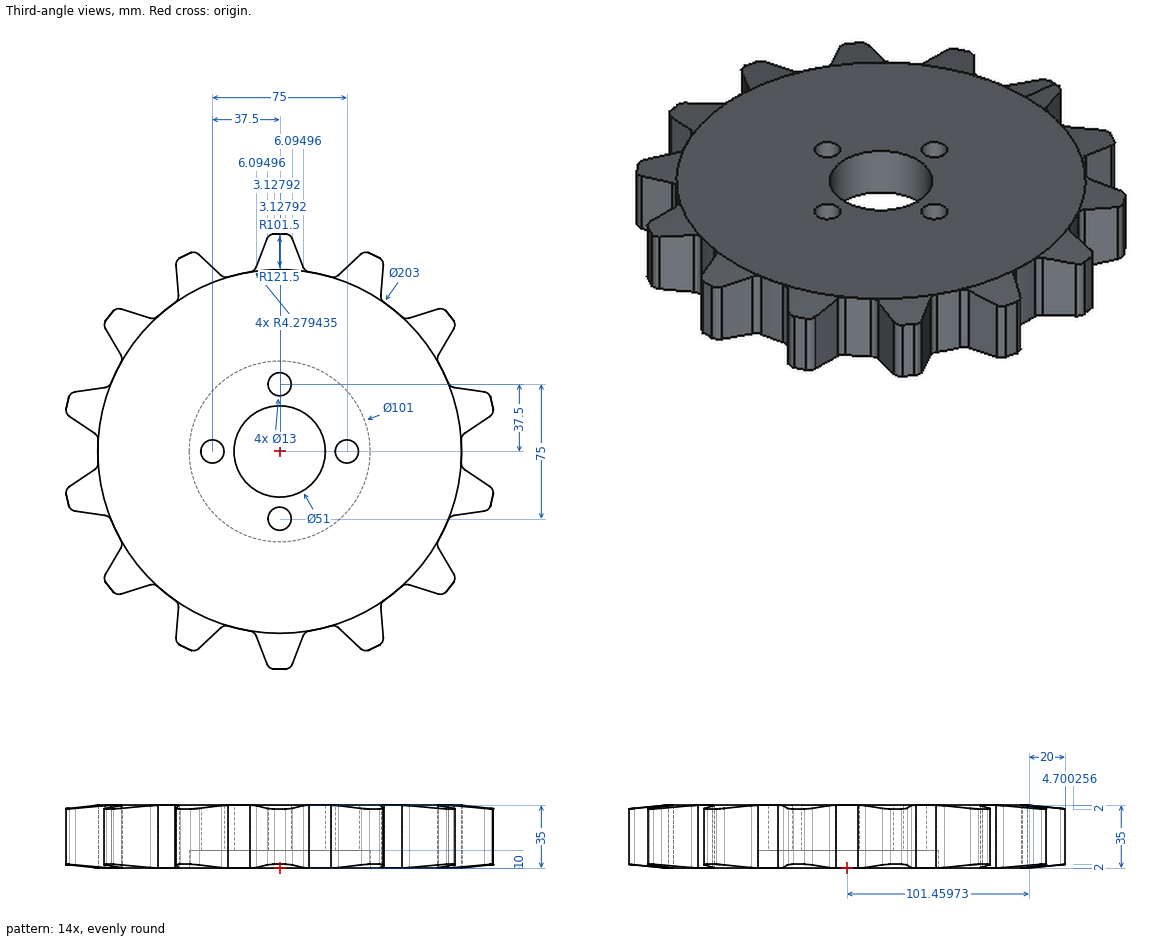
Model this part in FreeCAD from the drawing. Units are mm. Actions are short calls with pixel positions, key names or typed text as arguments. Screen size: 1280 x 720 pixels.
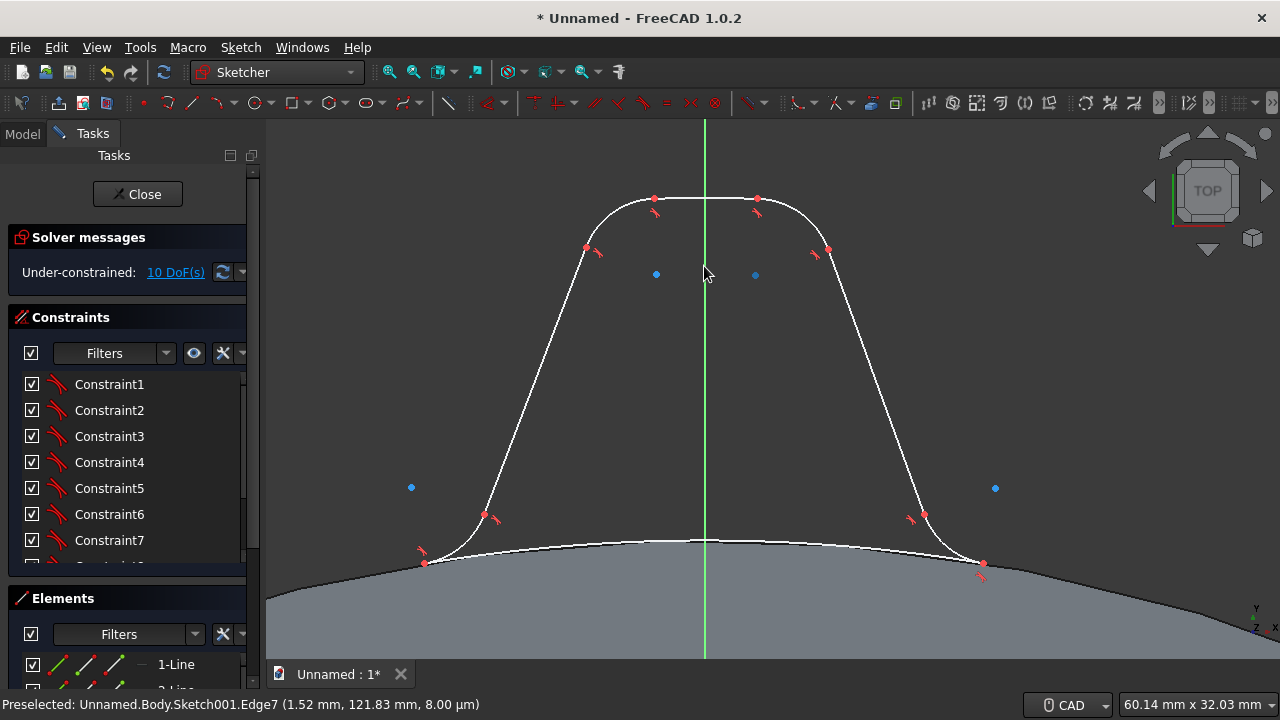
click(472, 536)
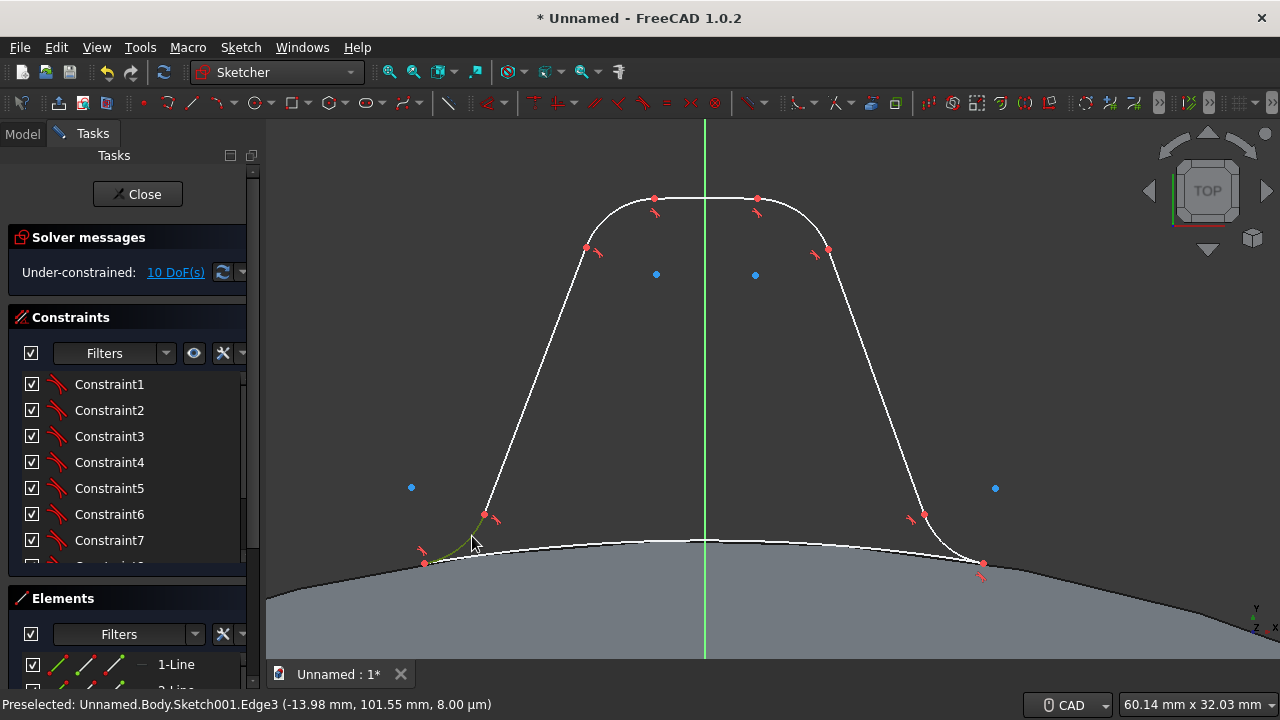
click(936, 535)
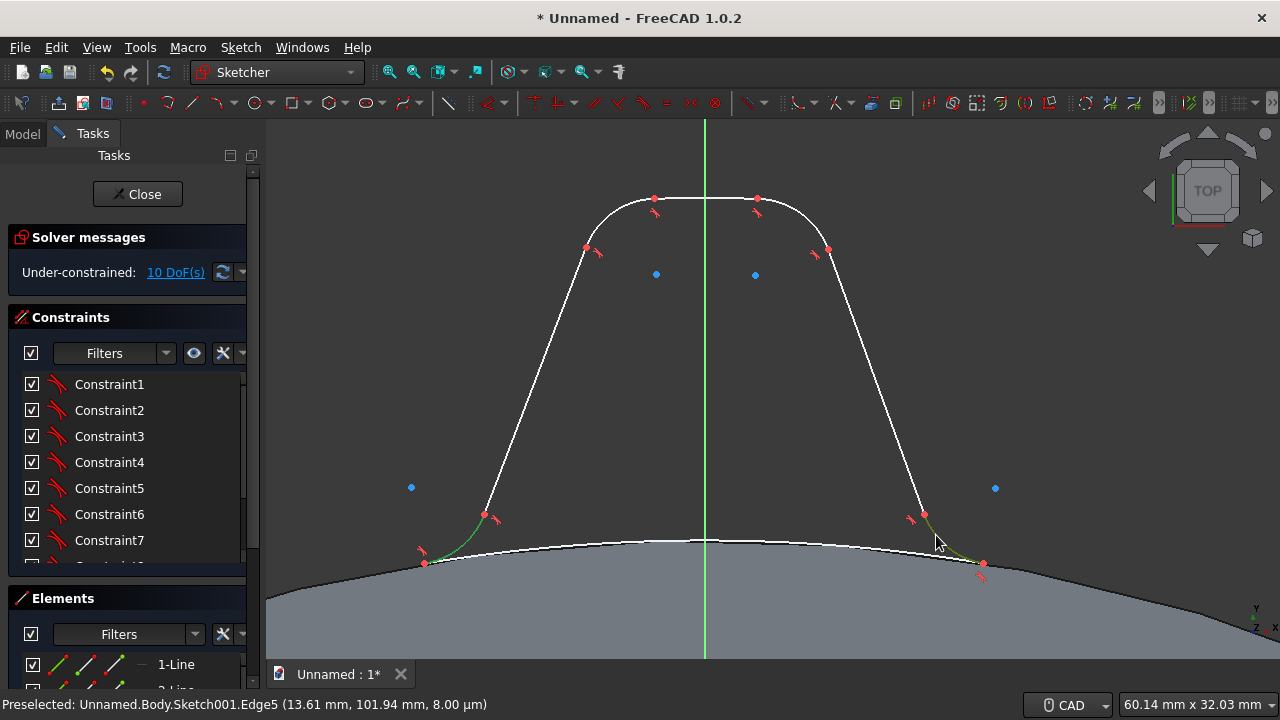
click(814, 226)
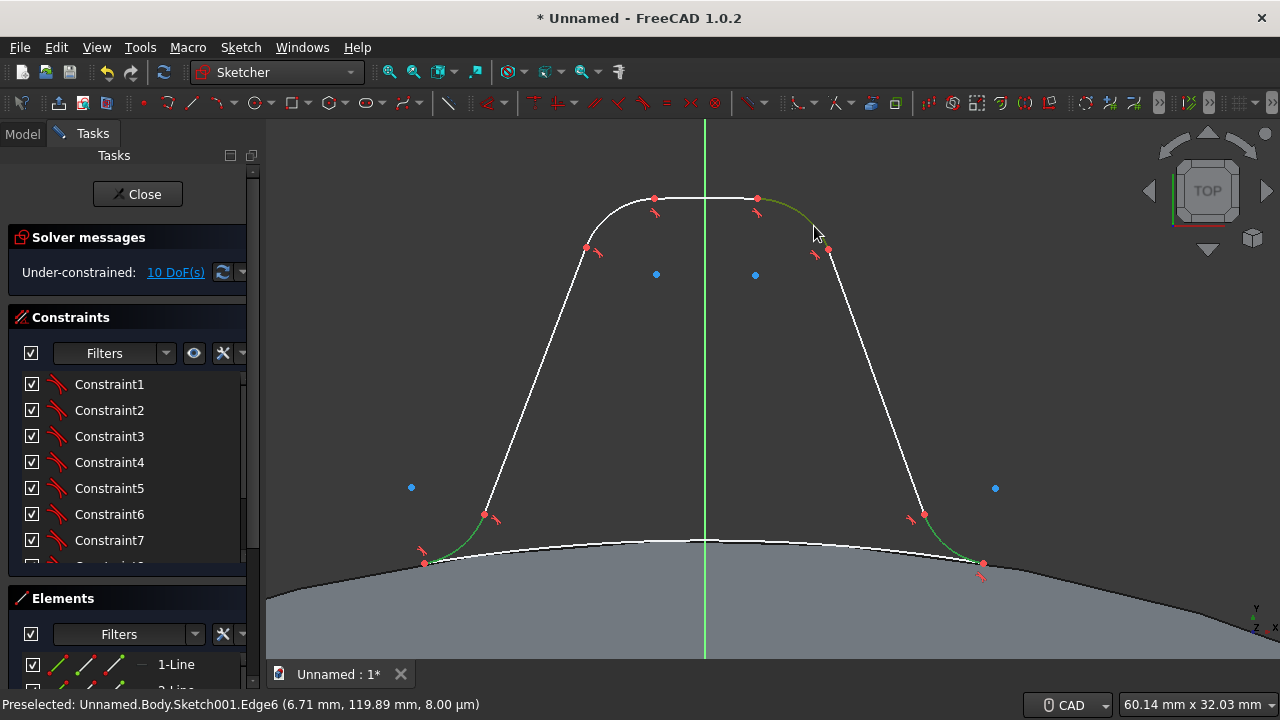
click(629, 204)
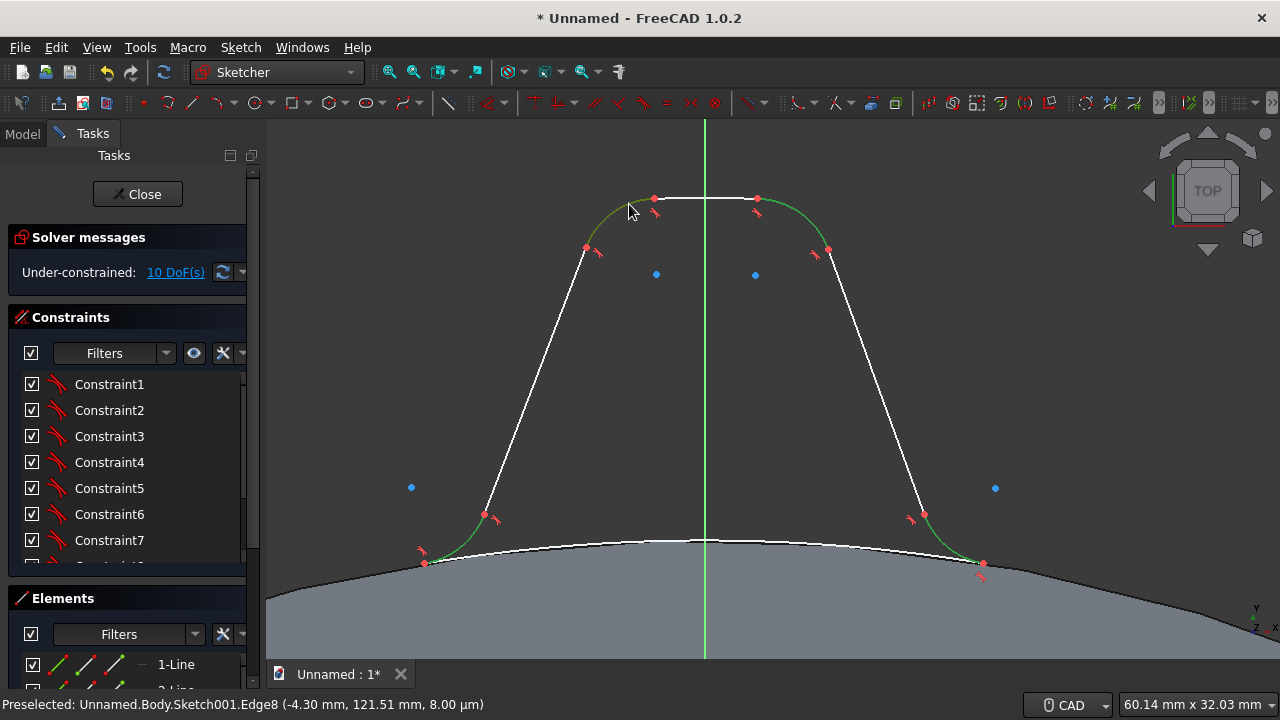
click(668, 104)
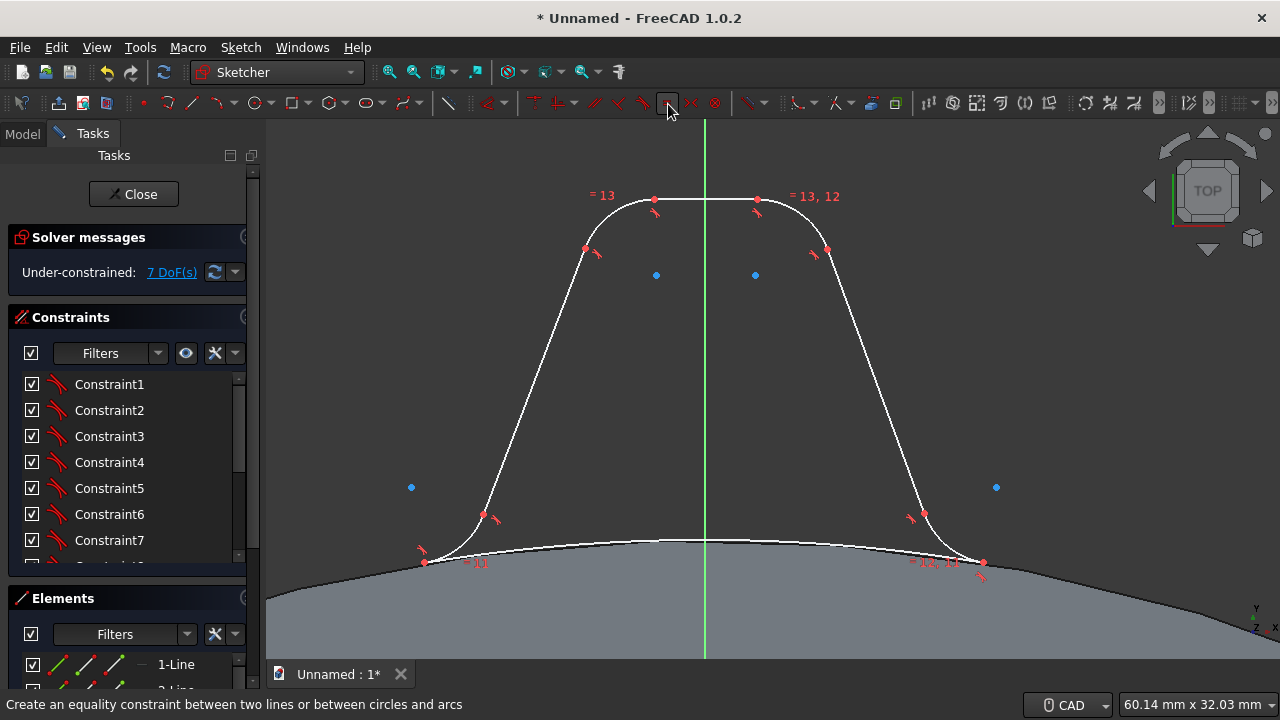
click(472, 535)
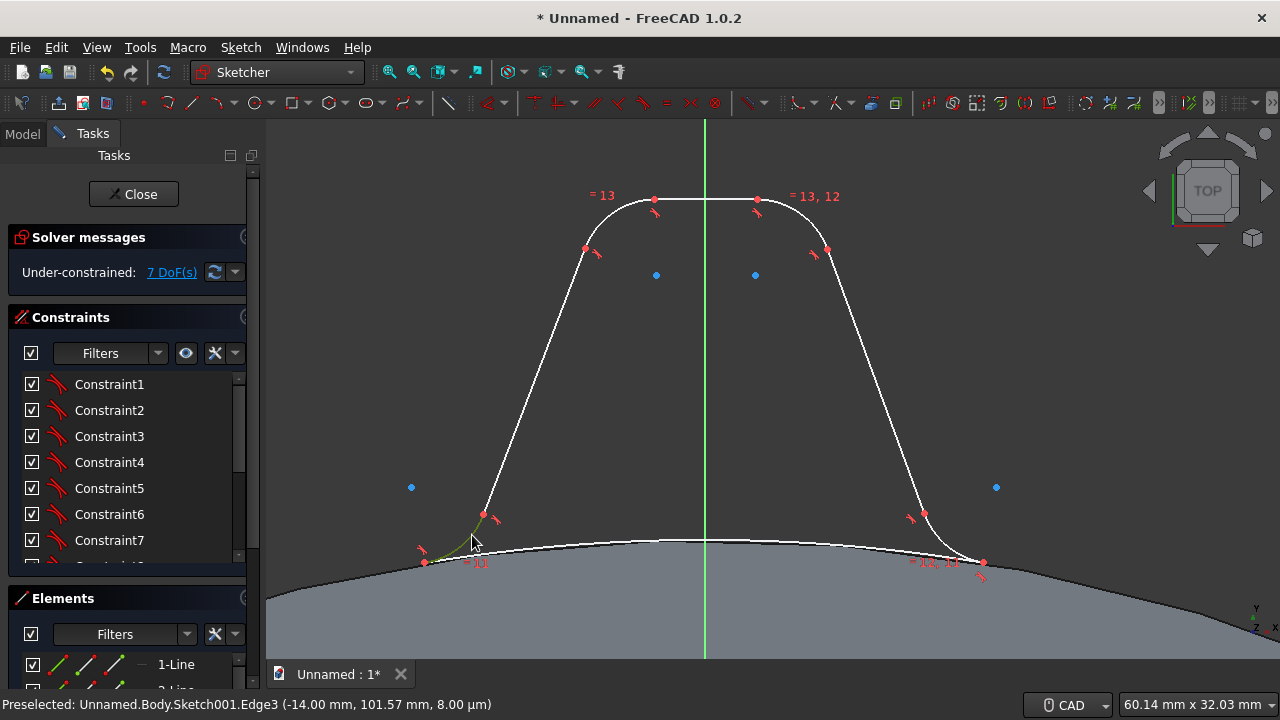
click(506, 104)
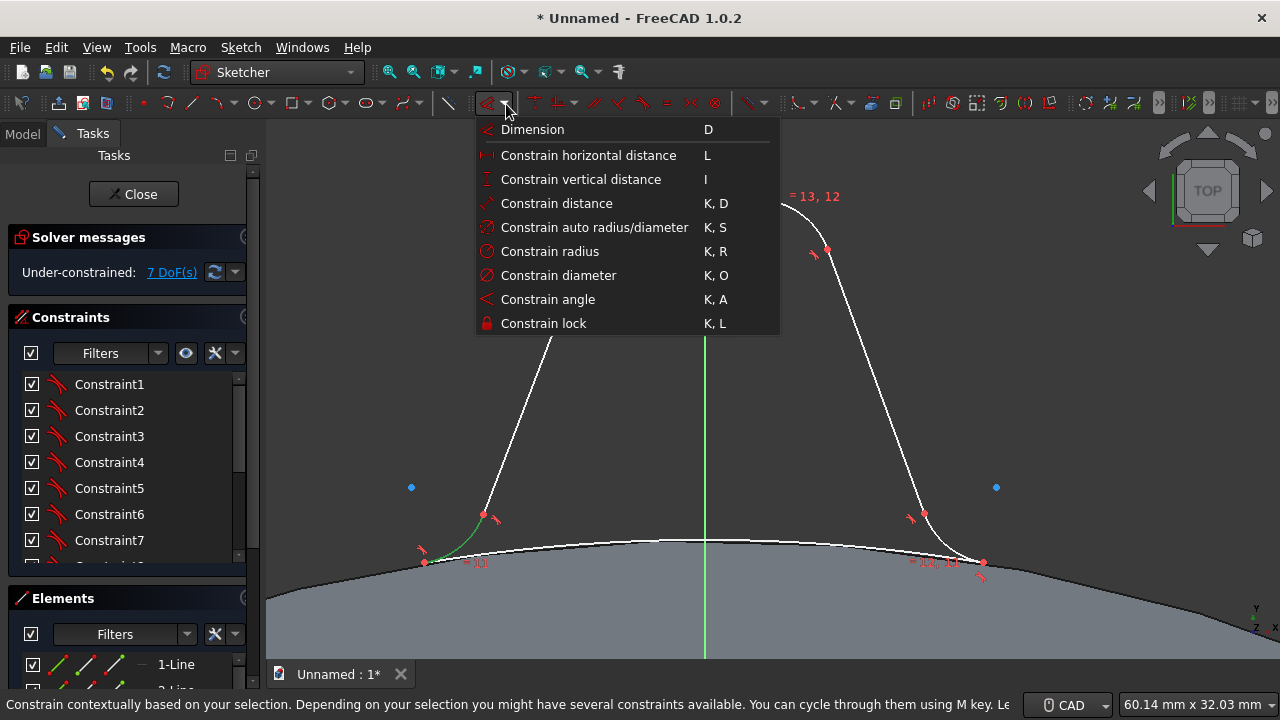
click(628, 251)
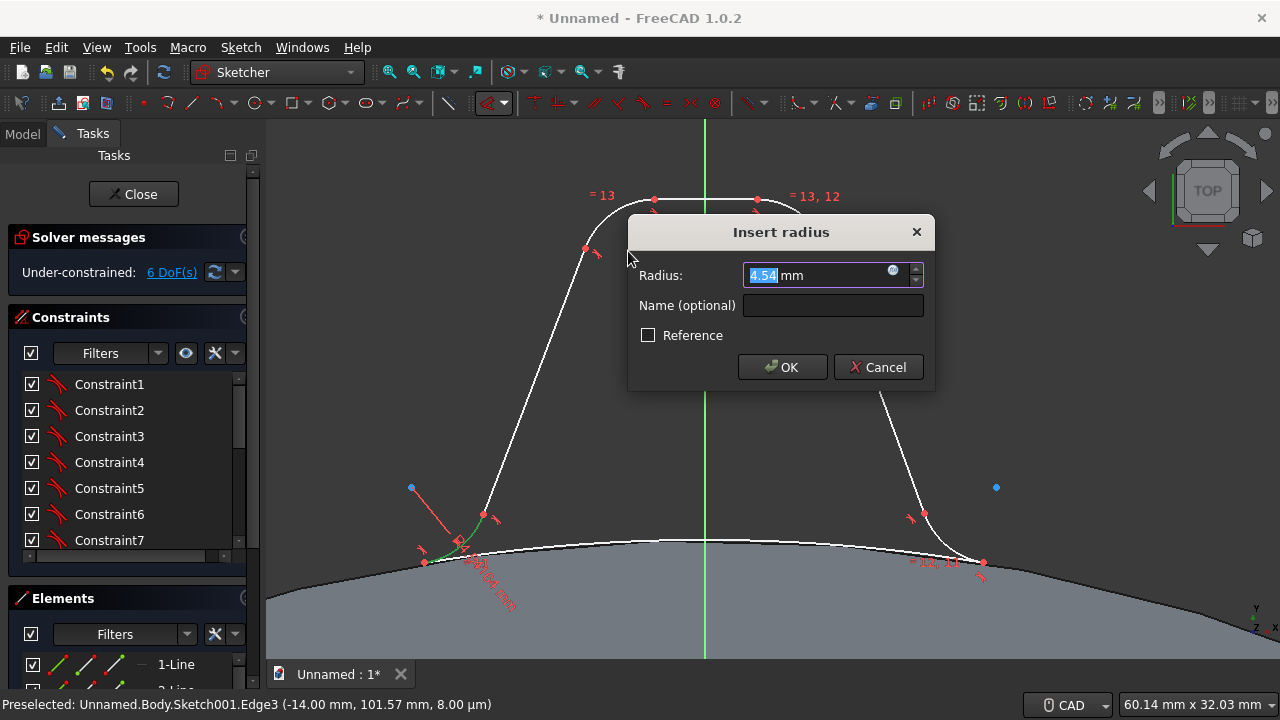
text(4.279435)
key(Return)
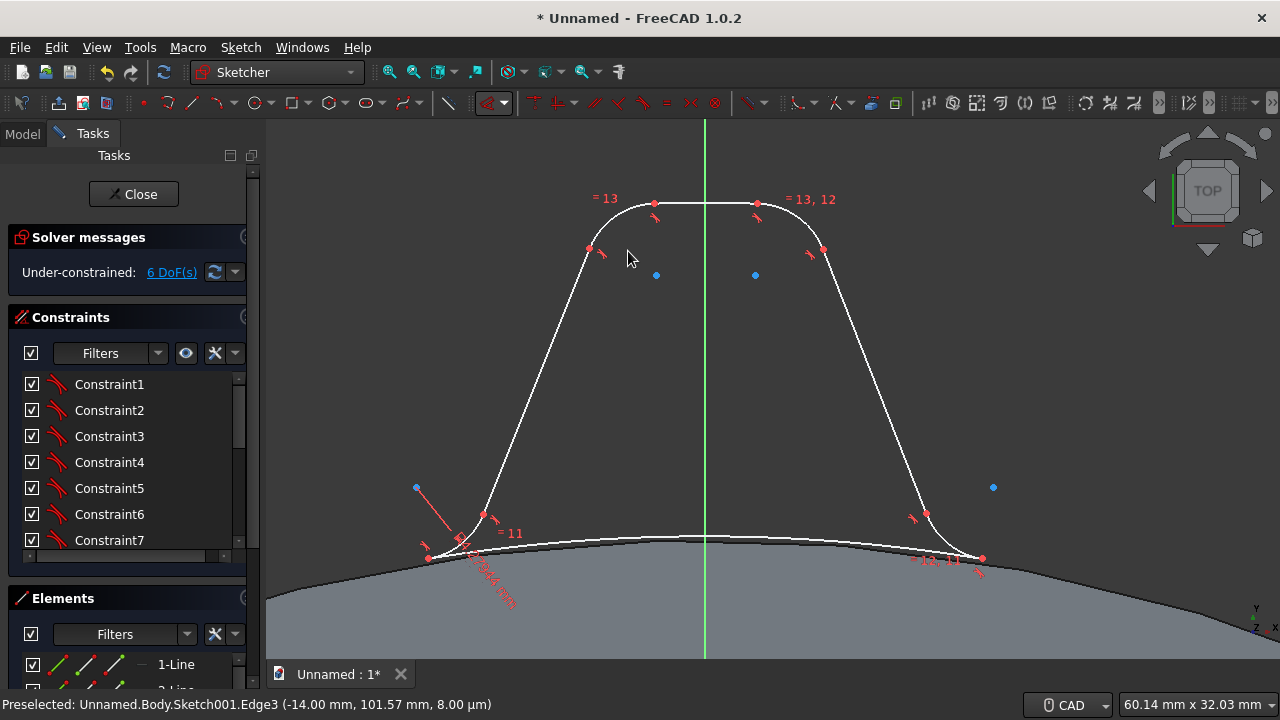
click(816, 540)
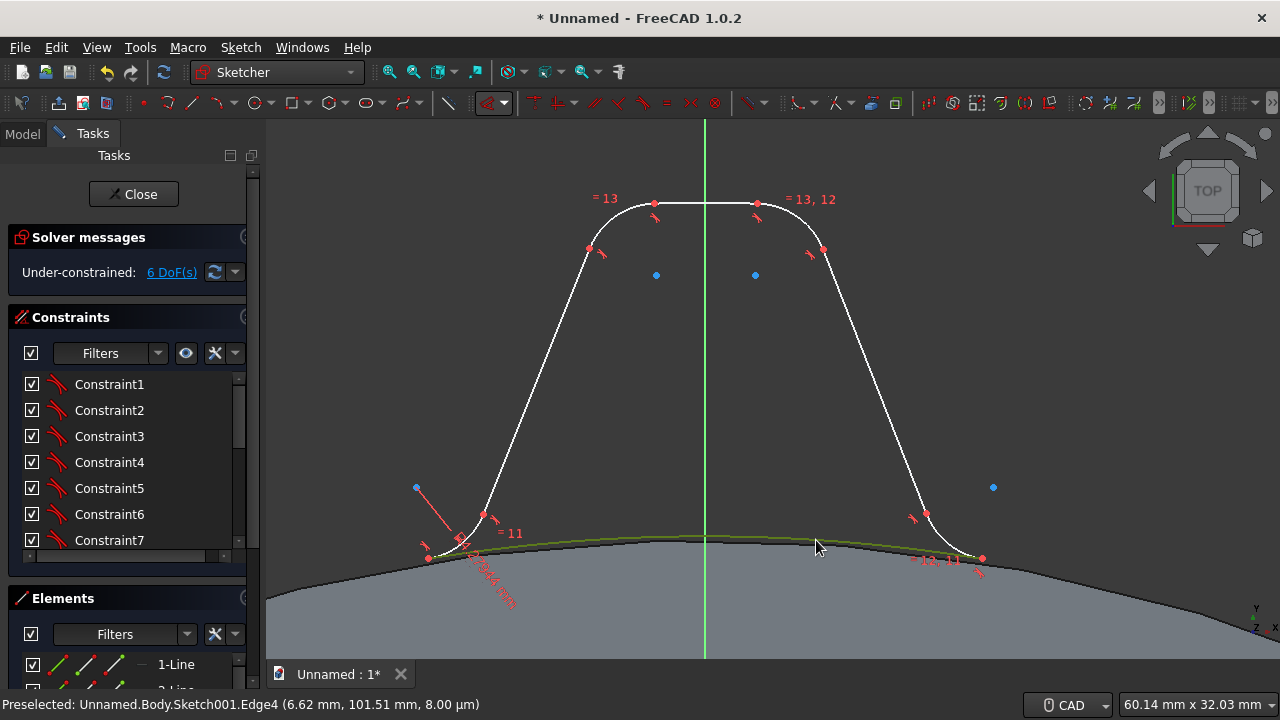
click(506, 104)